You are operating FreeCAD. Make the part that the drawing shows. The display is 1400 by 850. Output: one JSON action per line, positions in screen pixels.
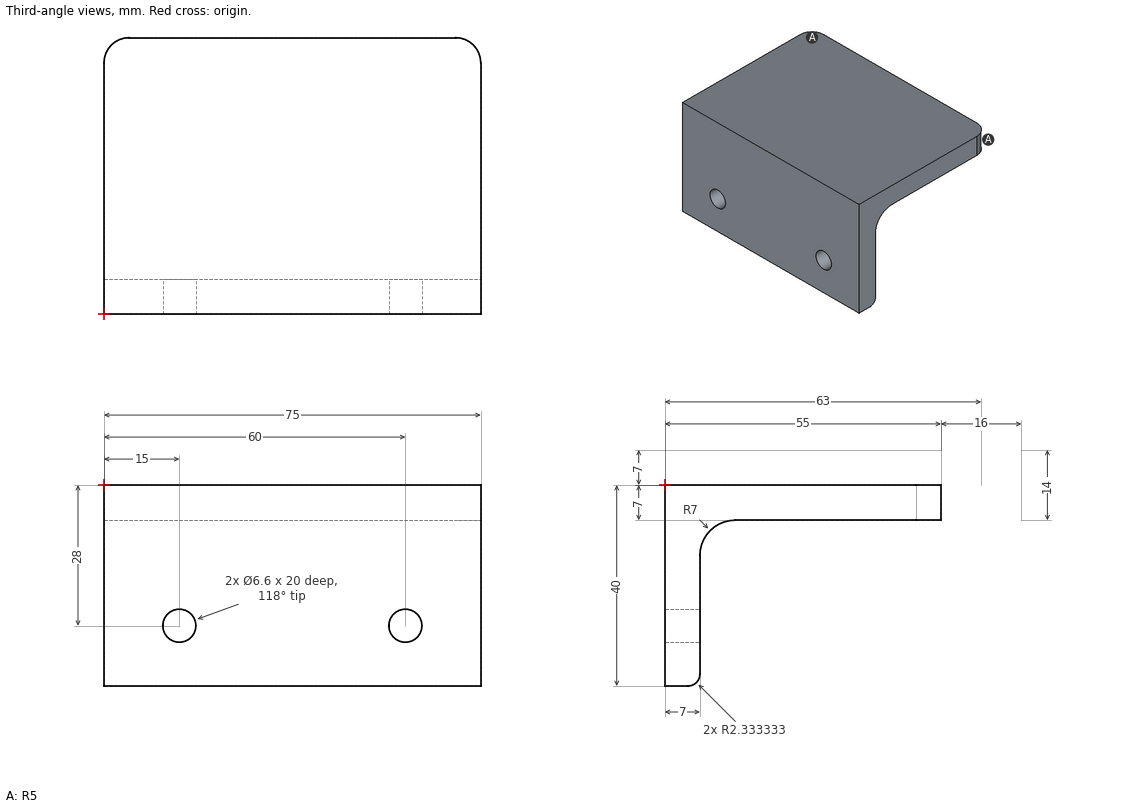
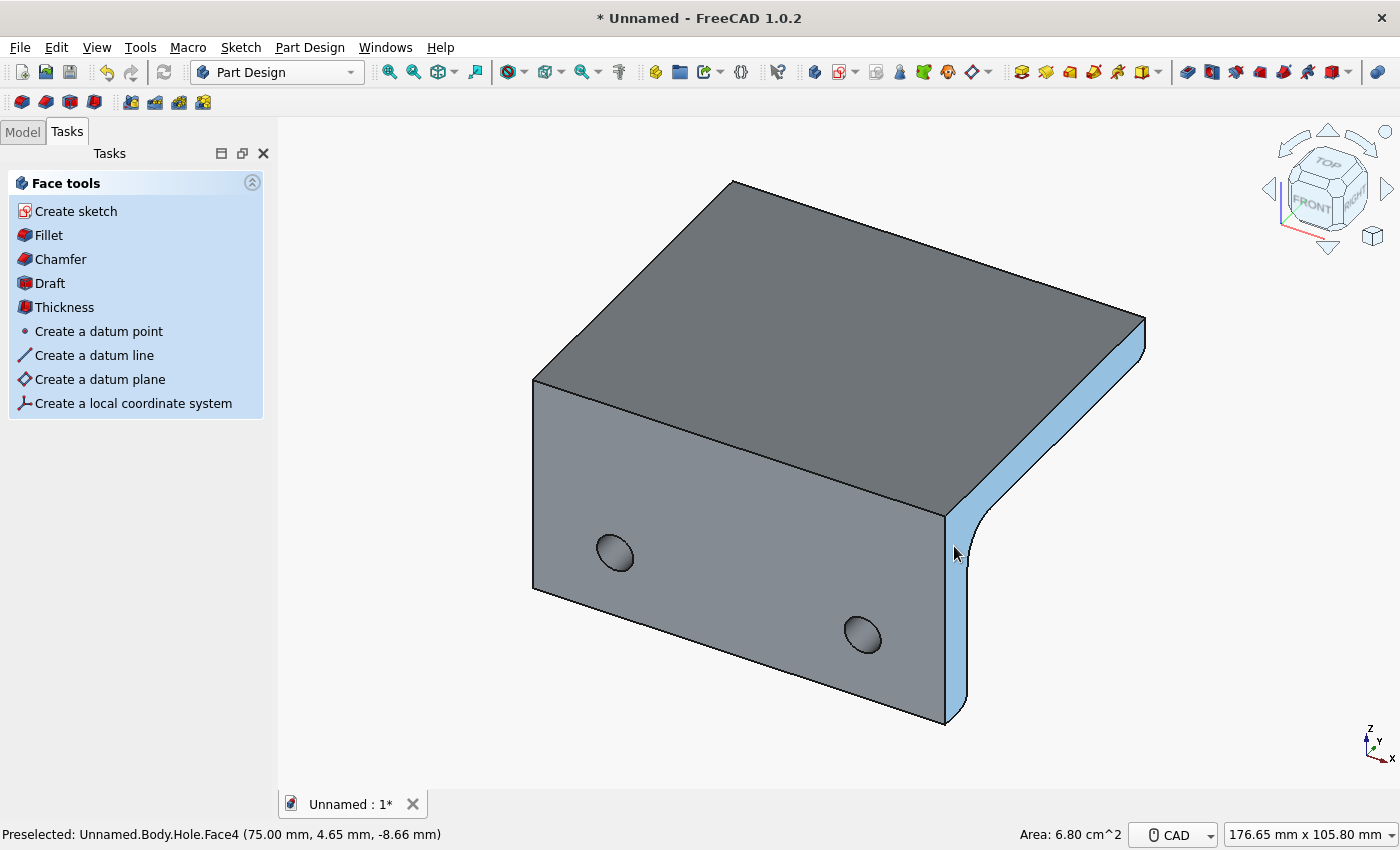
{"action": "left_click", "coordinate": [840, 72]}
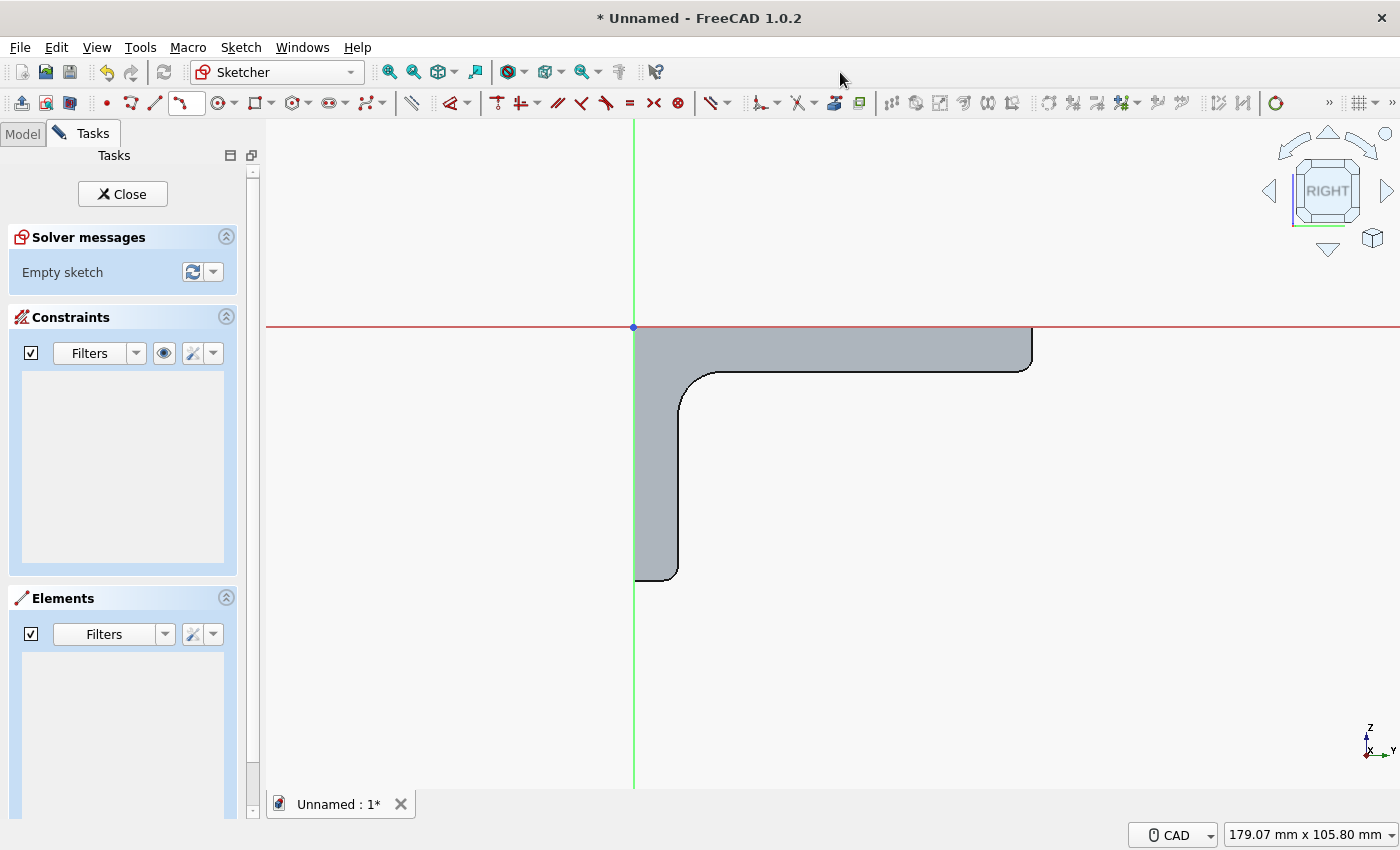
{"action": "scroll", "coordinate": [1100, 295], "scroll_direction": "up", "scroll_amount": 8}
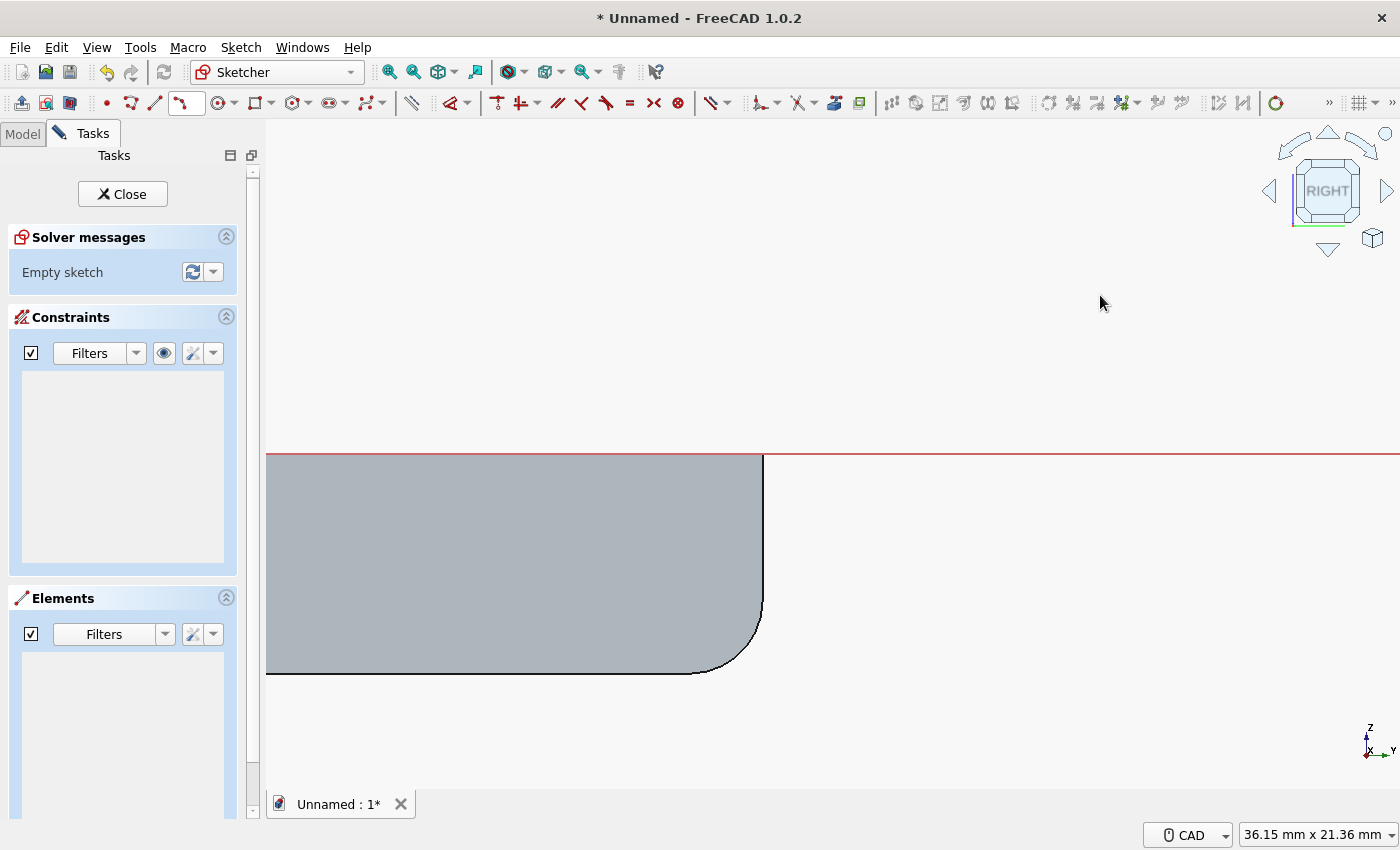
{"action": "left_click", "coordinate": [256, 104]}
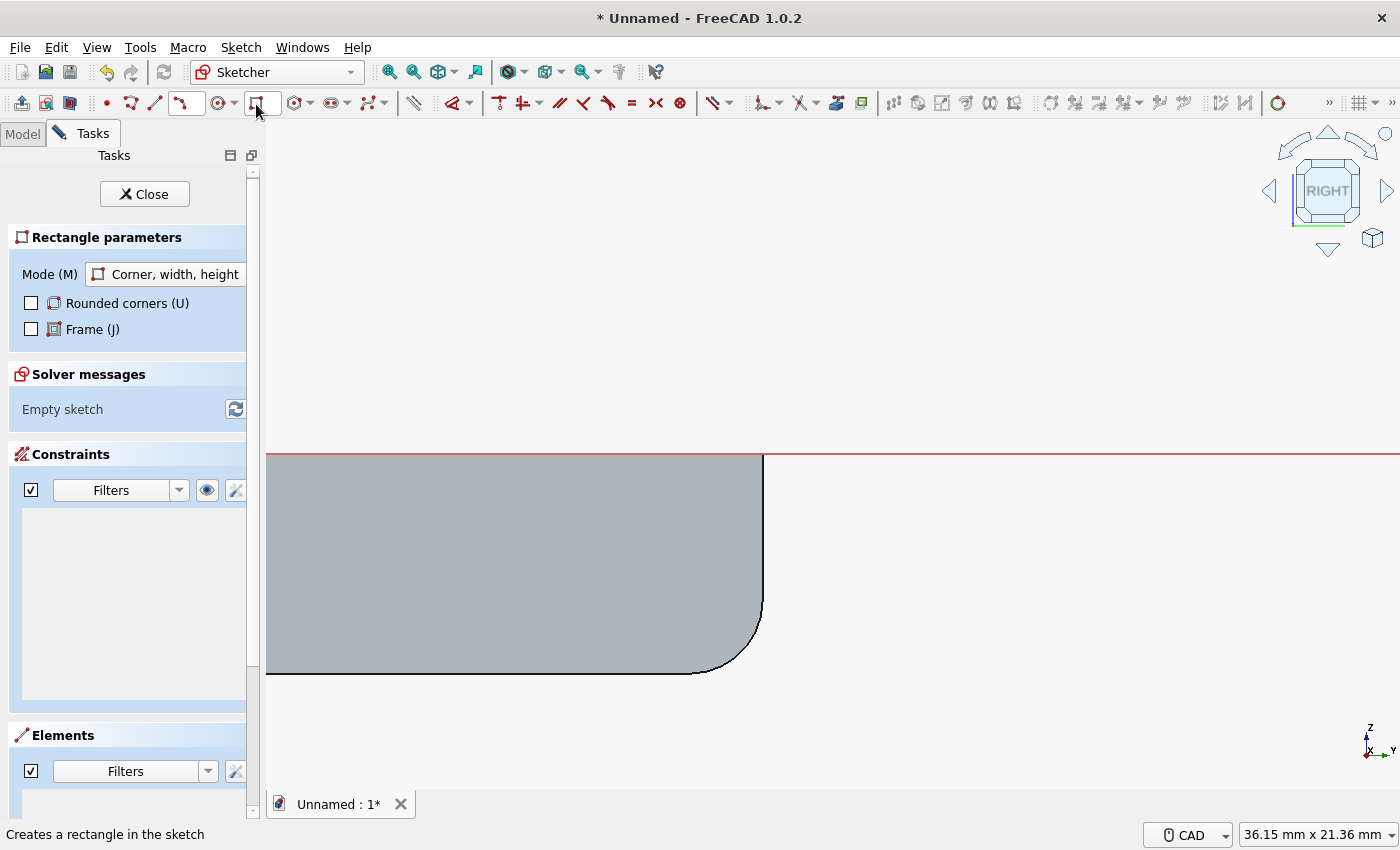
{"action": "left_click", "coordinate": [512, 235]}
{"action": "mouse_move", "coordinate": [1014, 674]}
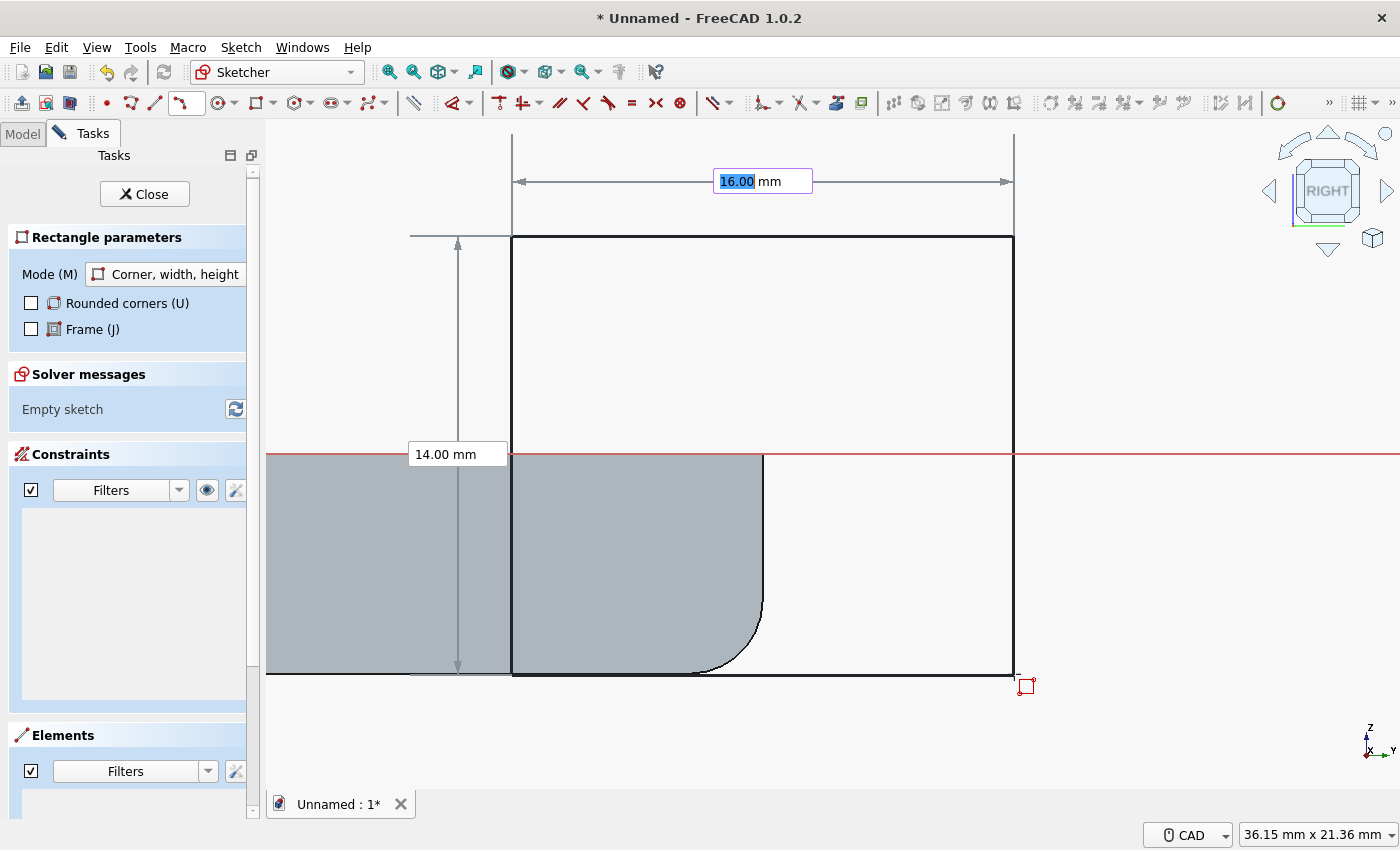
{"action": "type", "text": "16"}
{"action": "key", "text": "Tab"}
{"action": "type", "text": "14"}
{"action": "key", "text": "Return"}
{"action": "key", "text": "Escape"}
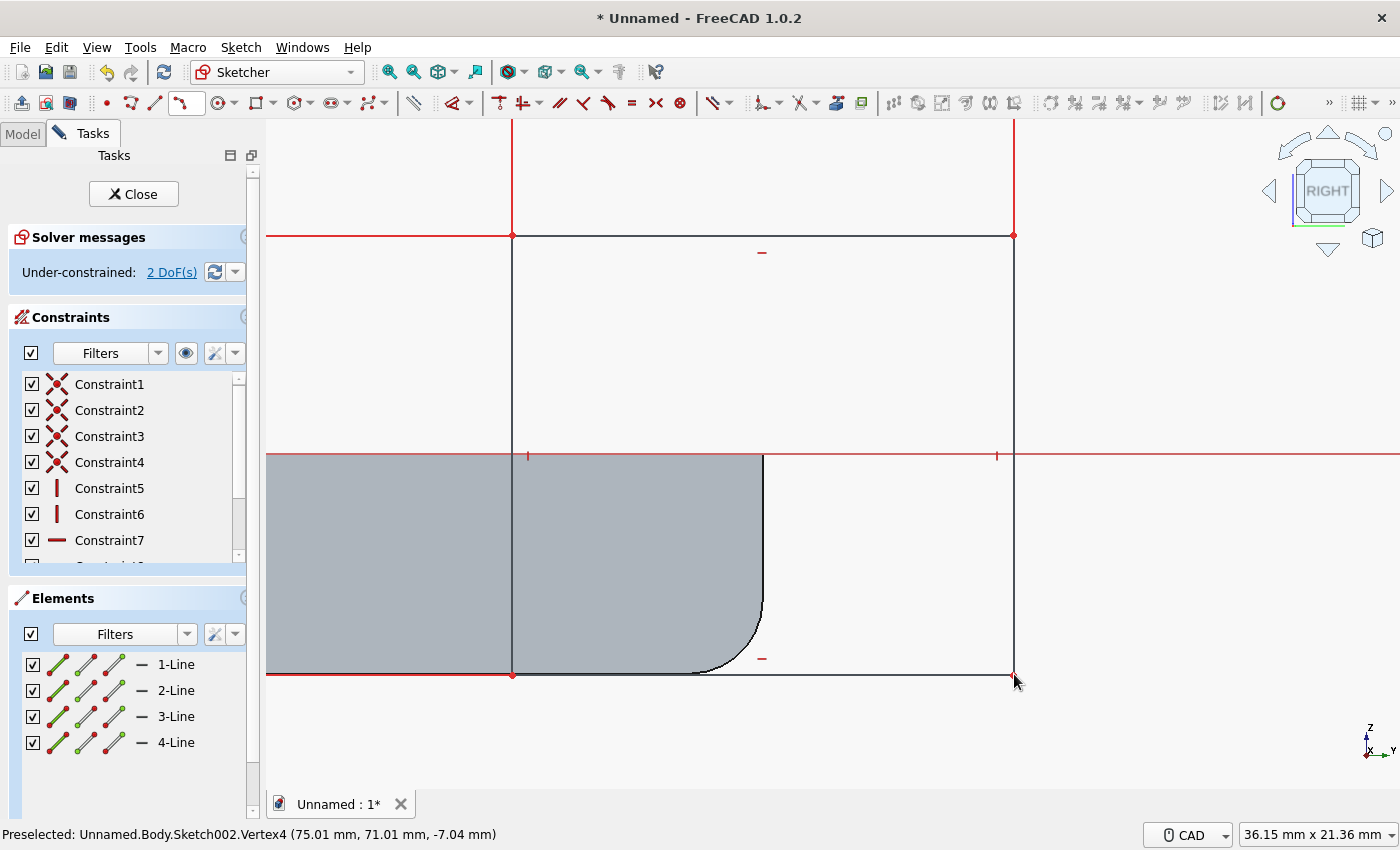
{"action": "key", "text": "d"}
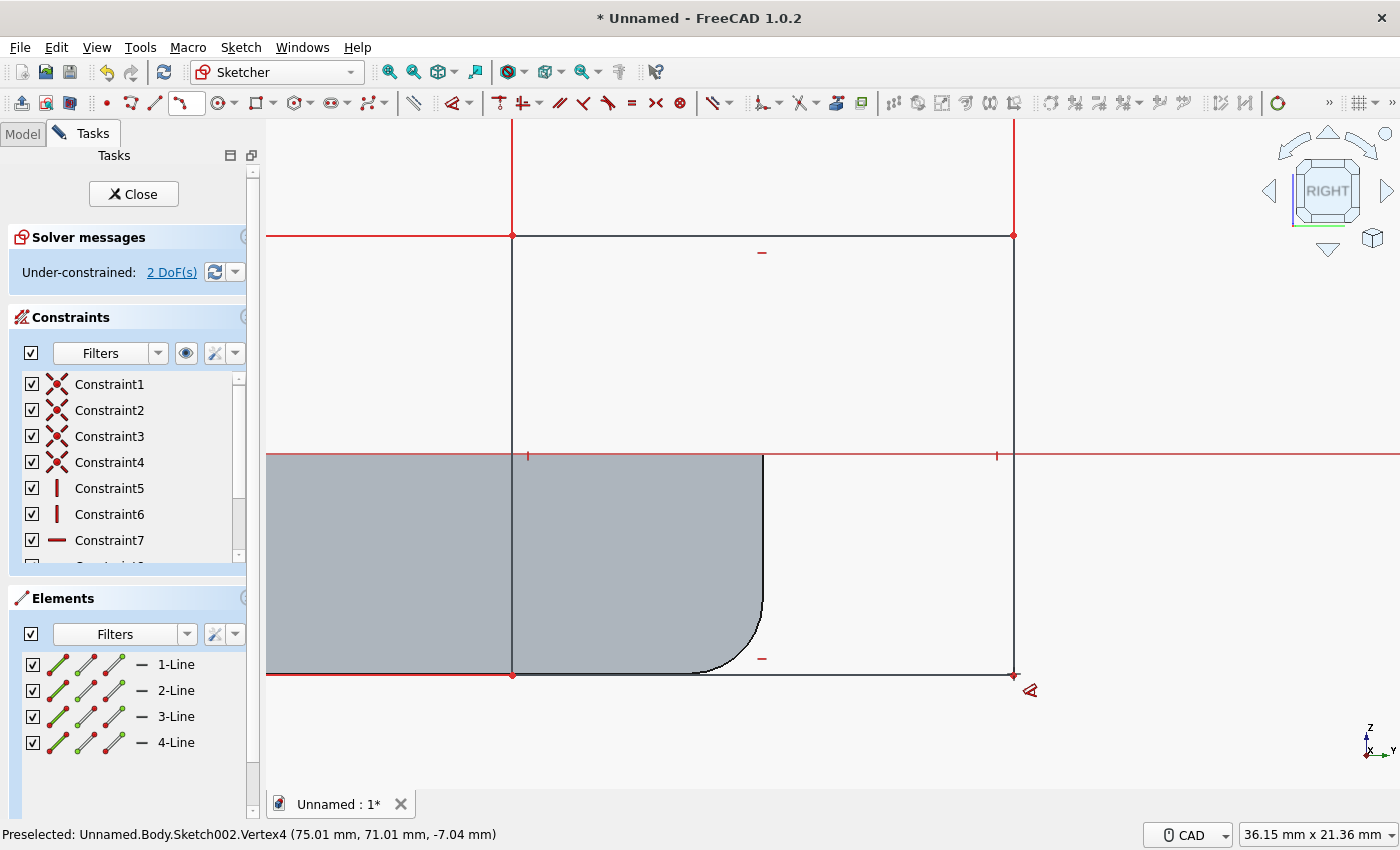
{"action": "left_click", "coordinate": [512, 236]}
{"action": "left_click", "coordinate": [546, 345]}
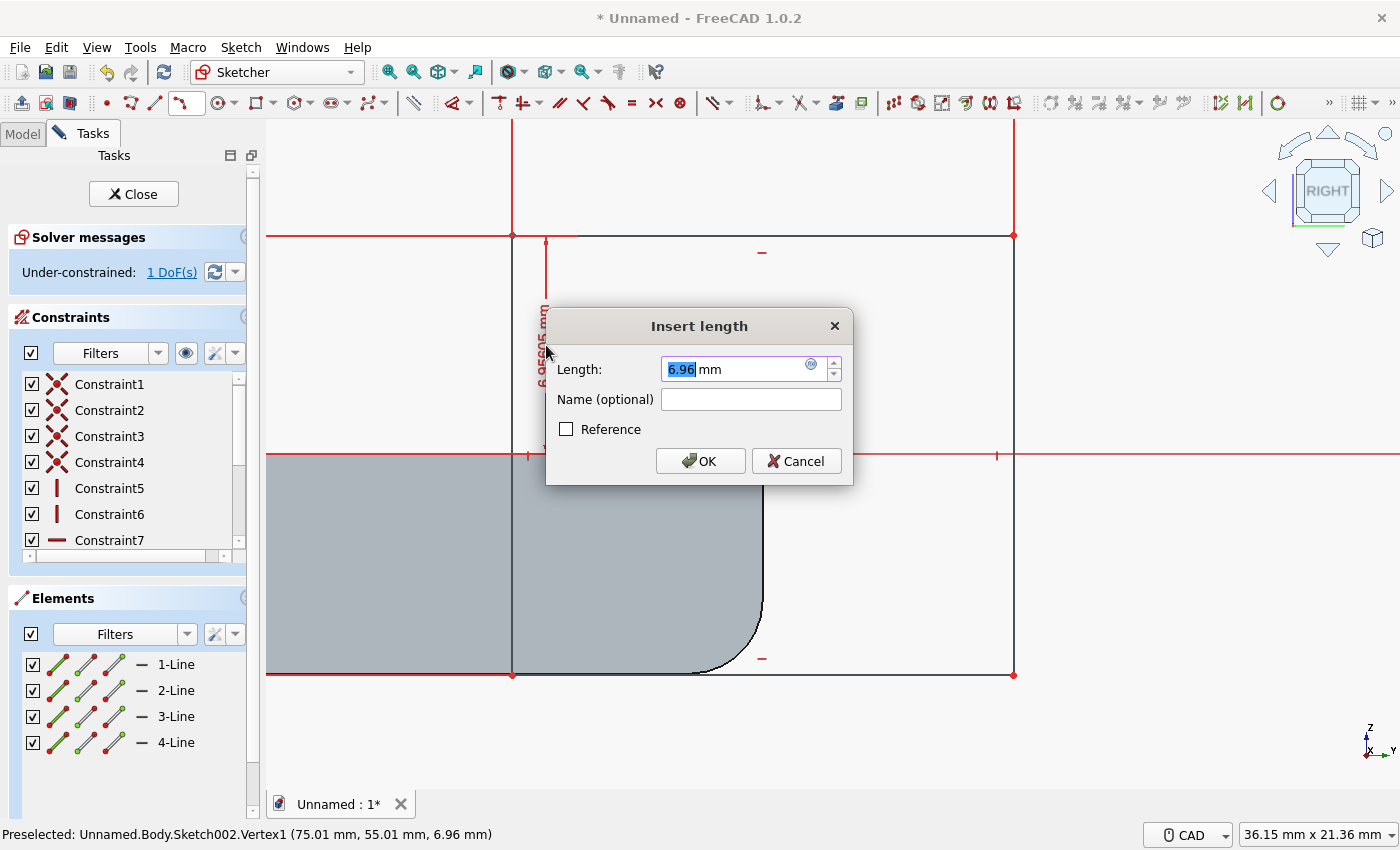
{"action": "type", "text": "7"}
{"action": "key", "text": "Return"}